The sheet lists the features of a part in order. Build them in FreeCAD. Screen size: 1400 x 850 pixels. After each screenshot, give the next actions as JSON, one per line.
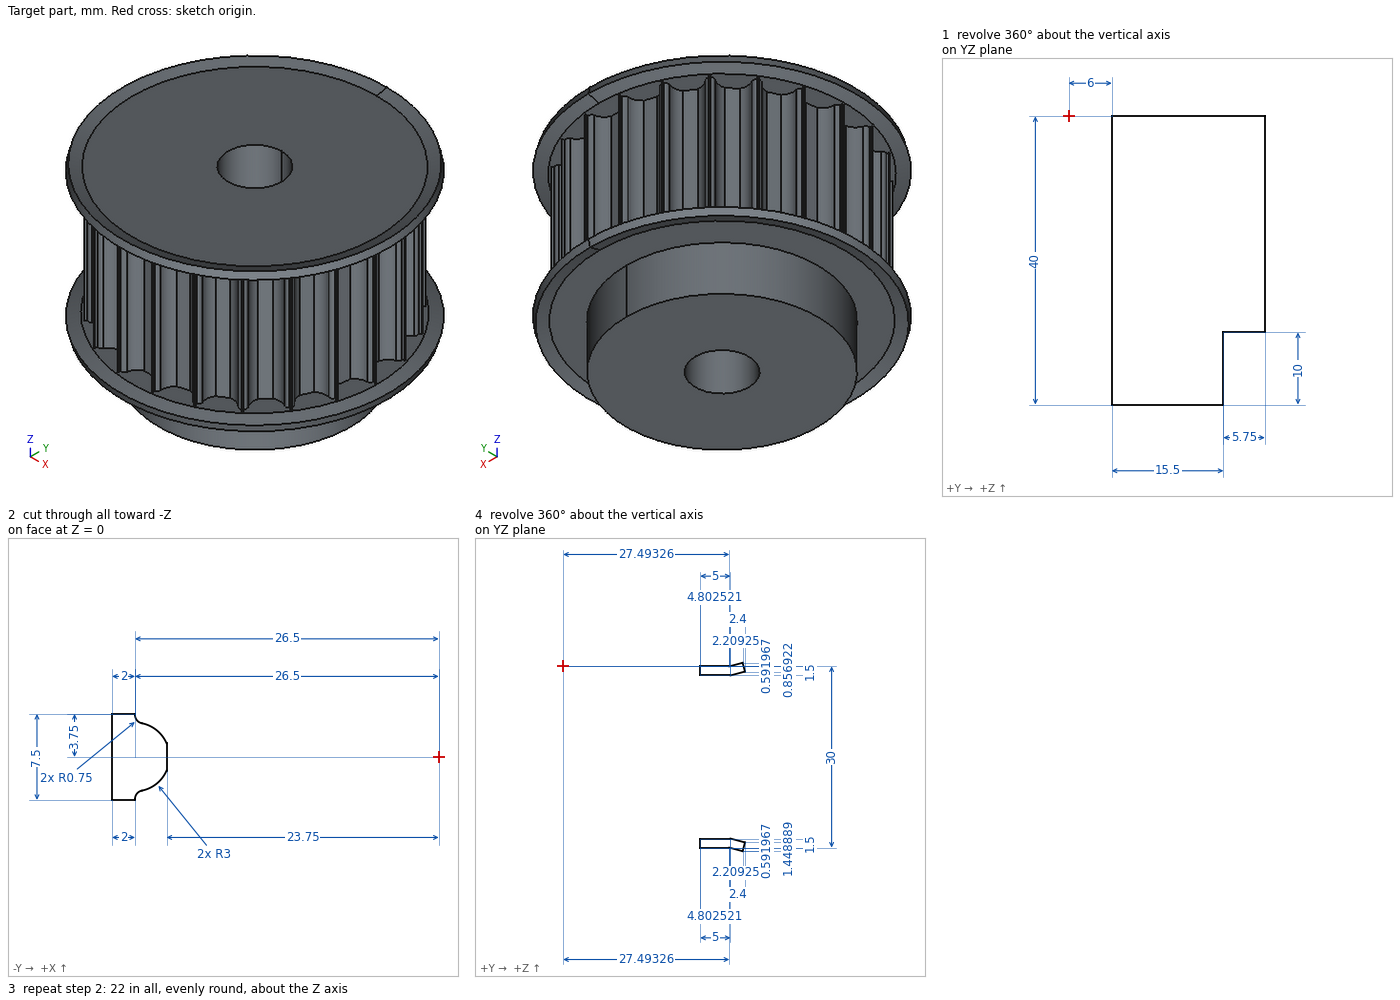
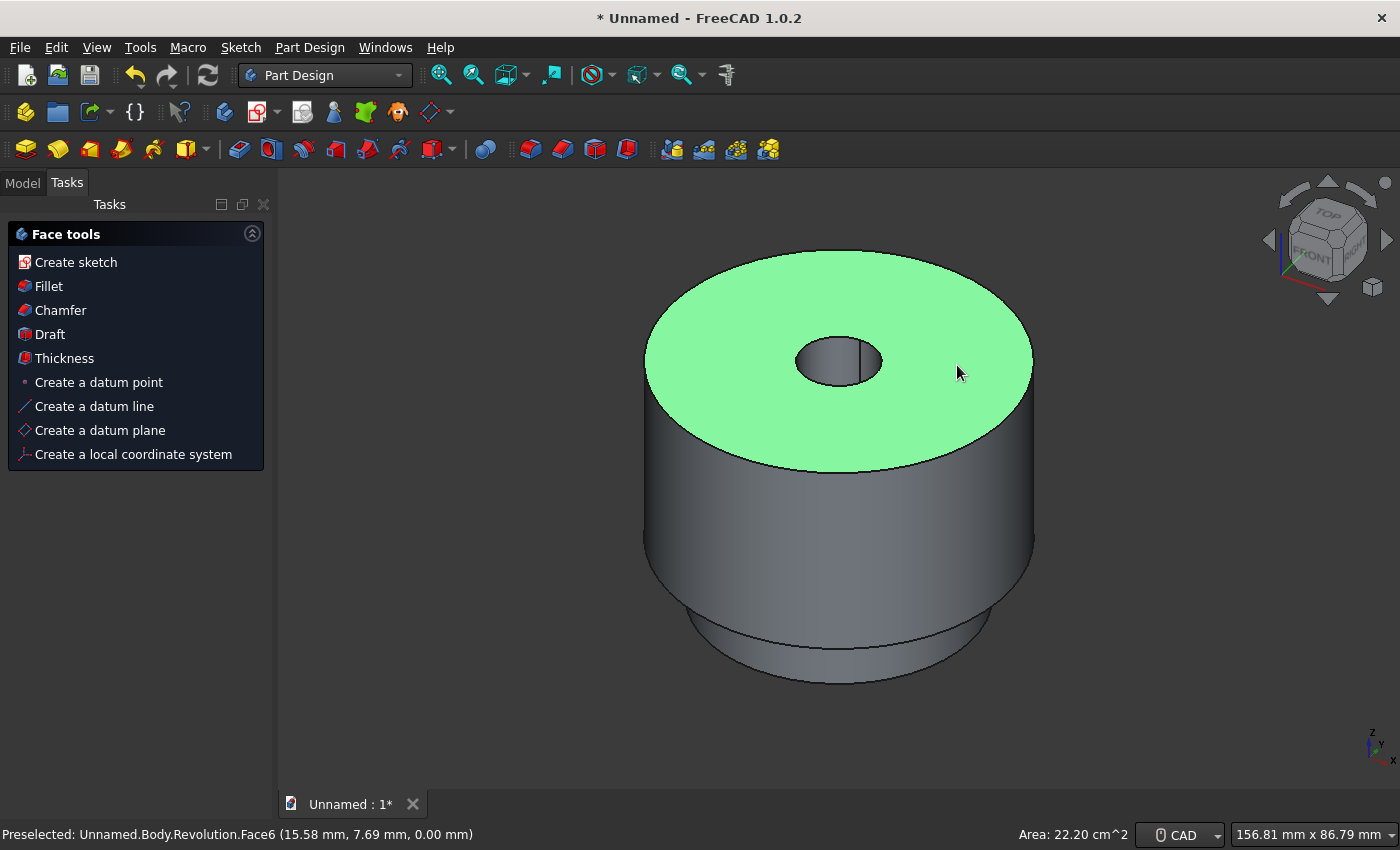
{"action": "left_click", "coordinate": [258, 112]}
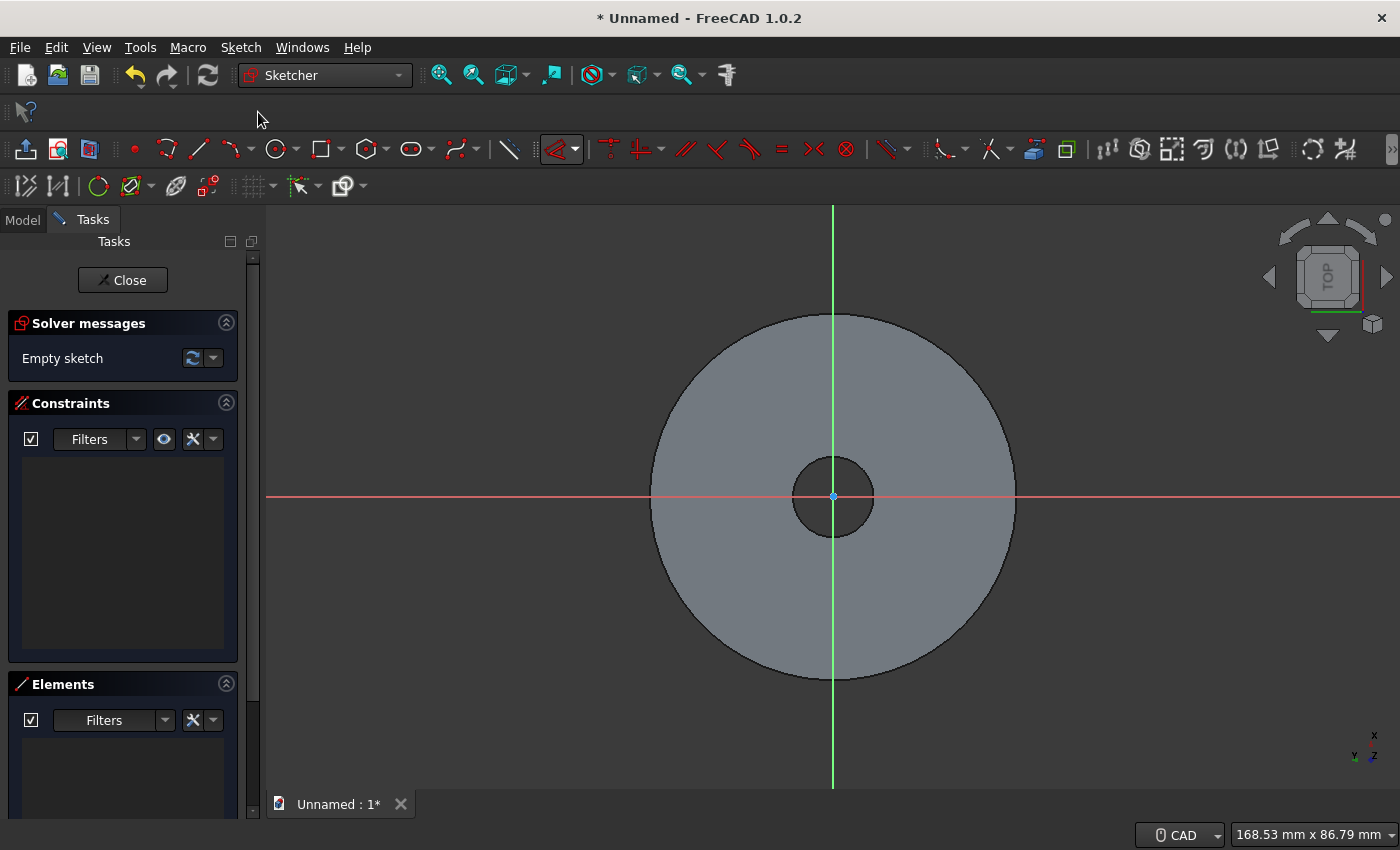
{"action": "scroll", "coordinate": [641, 497], "scroll_direction": "up", "scroll_amount": 10}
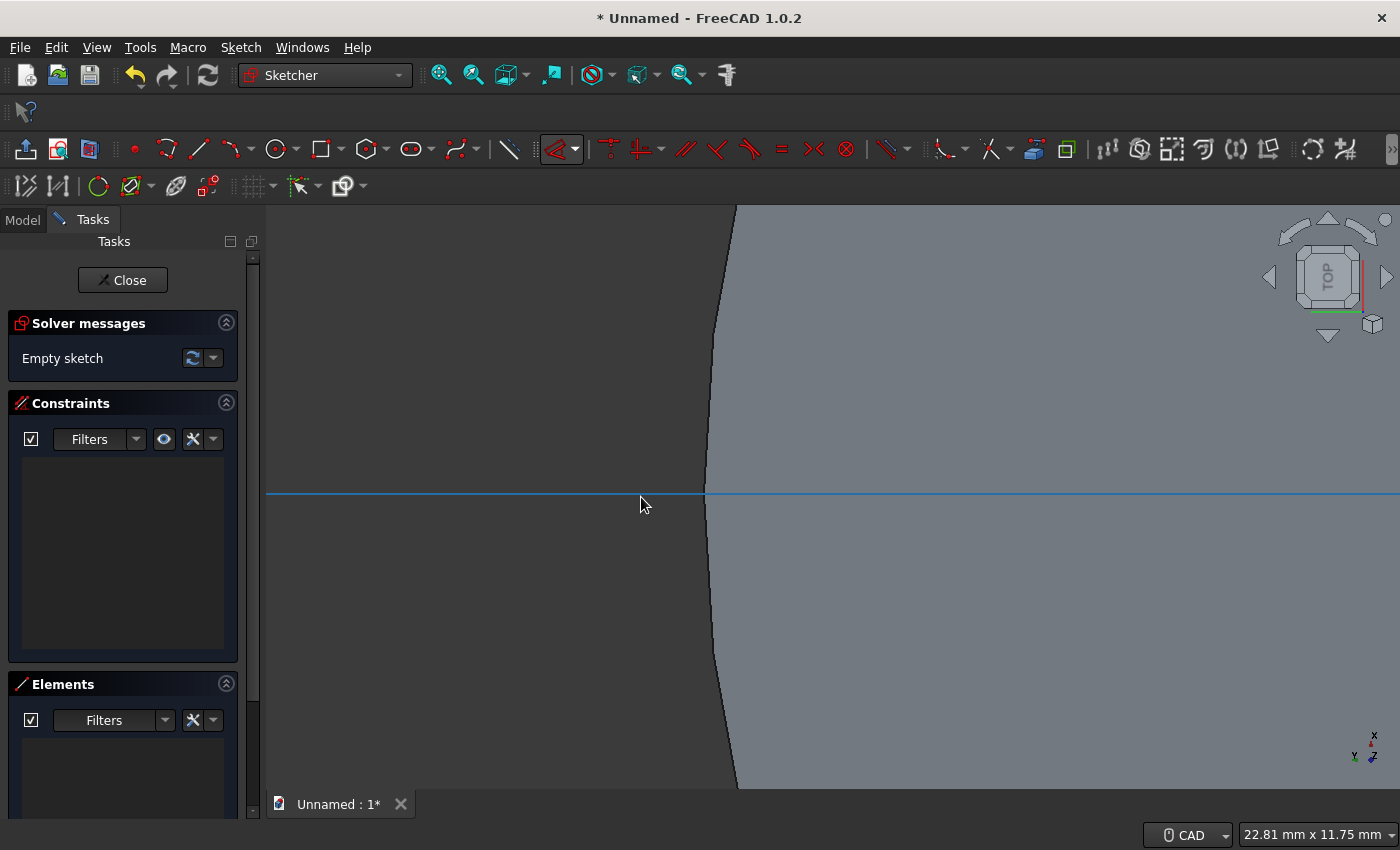
{"action": "left_click", "coordinate": [168, 150]}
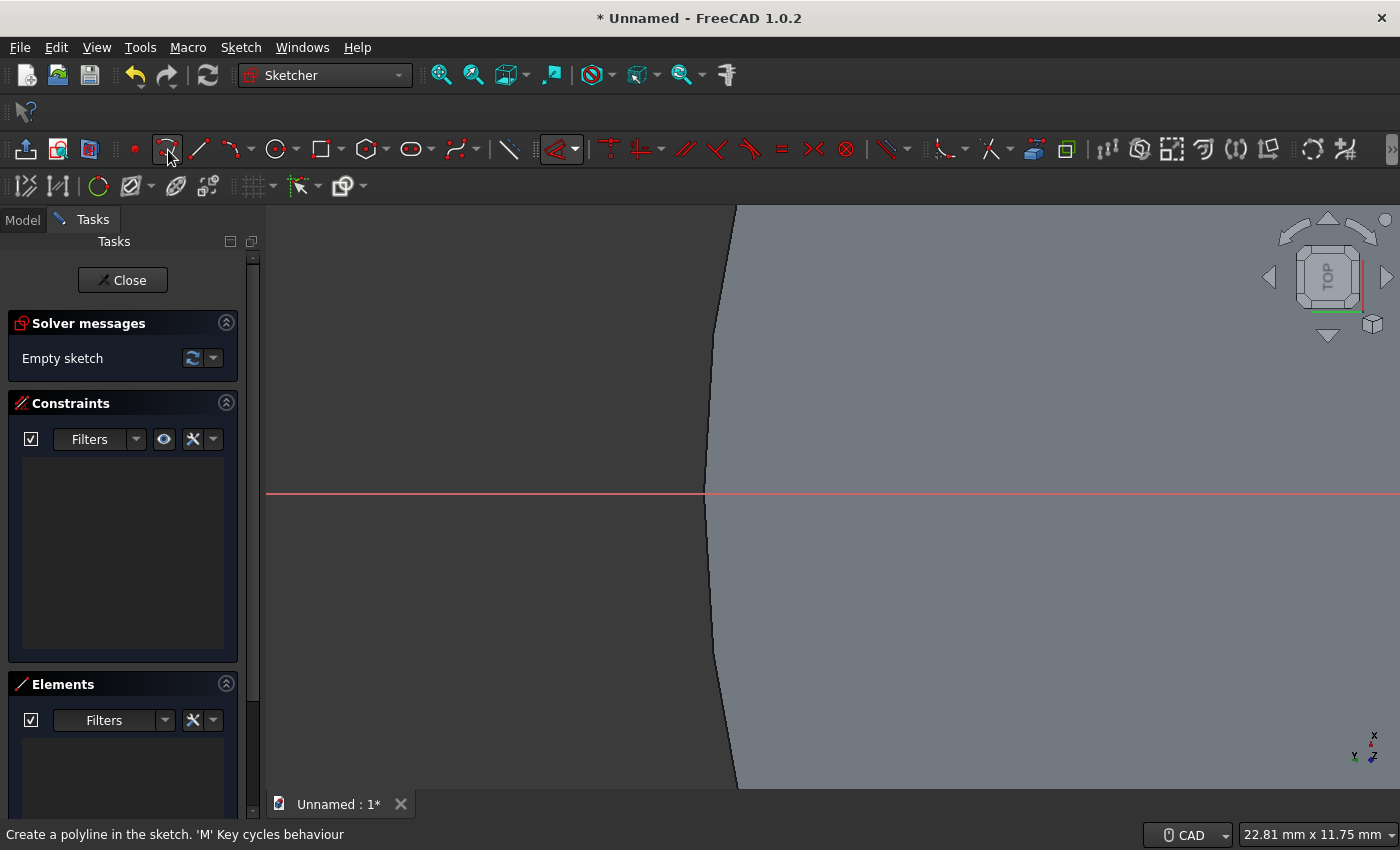
{"action": "left_click", "coordinate": [741, 311]}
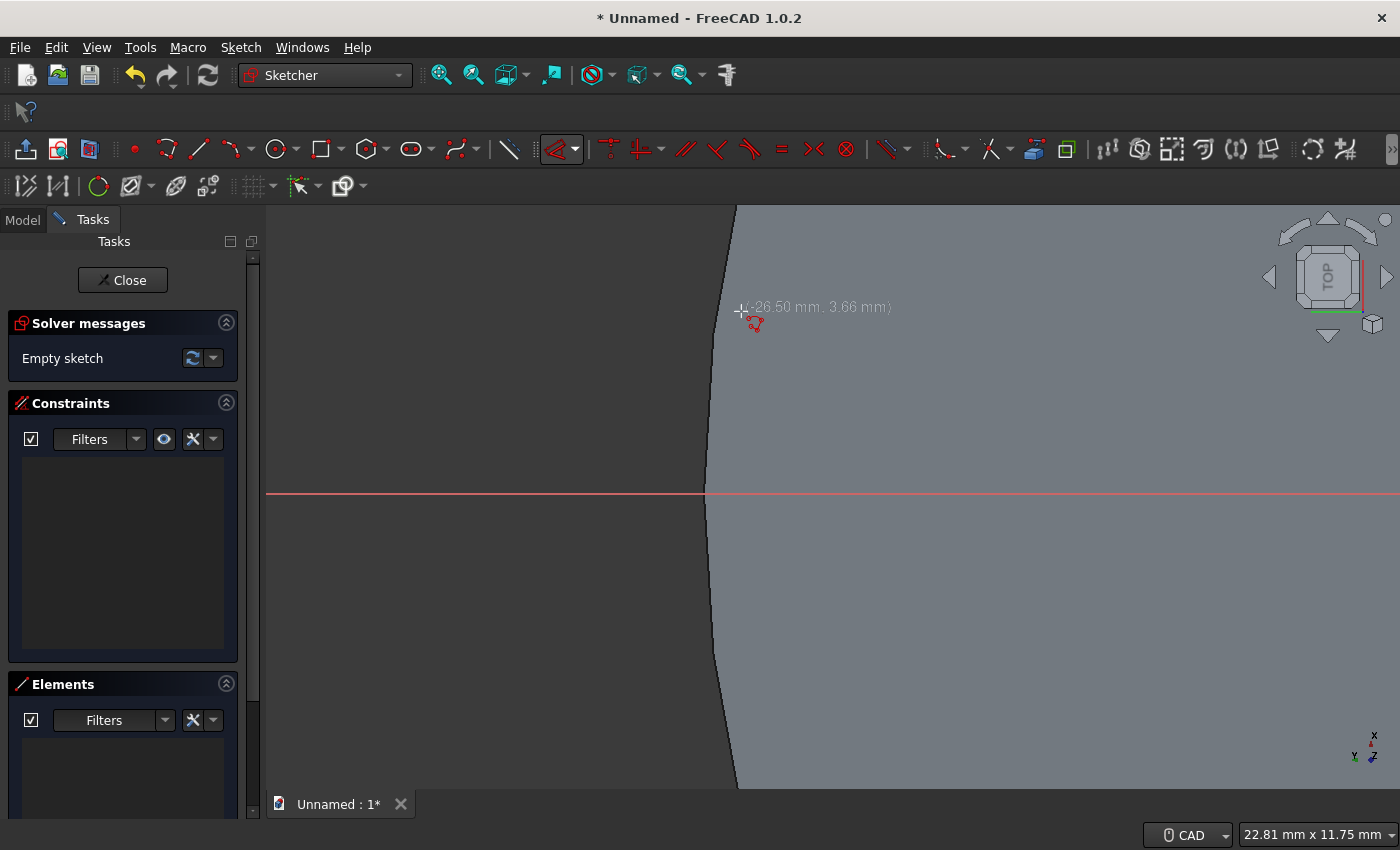
{"action": "scroll", "coordinate": [741, 307], "scroll_direction": "up", "scroll_amount": 8}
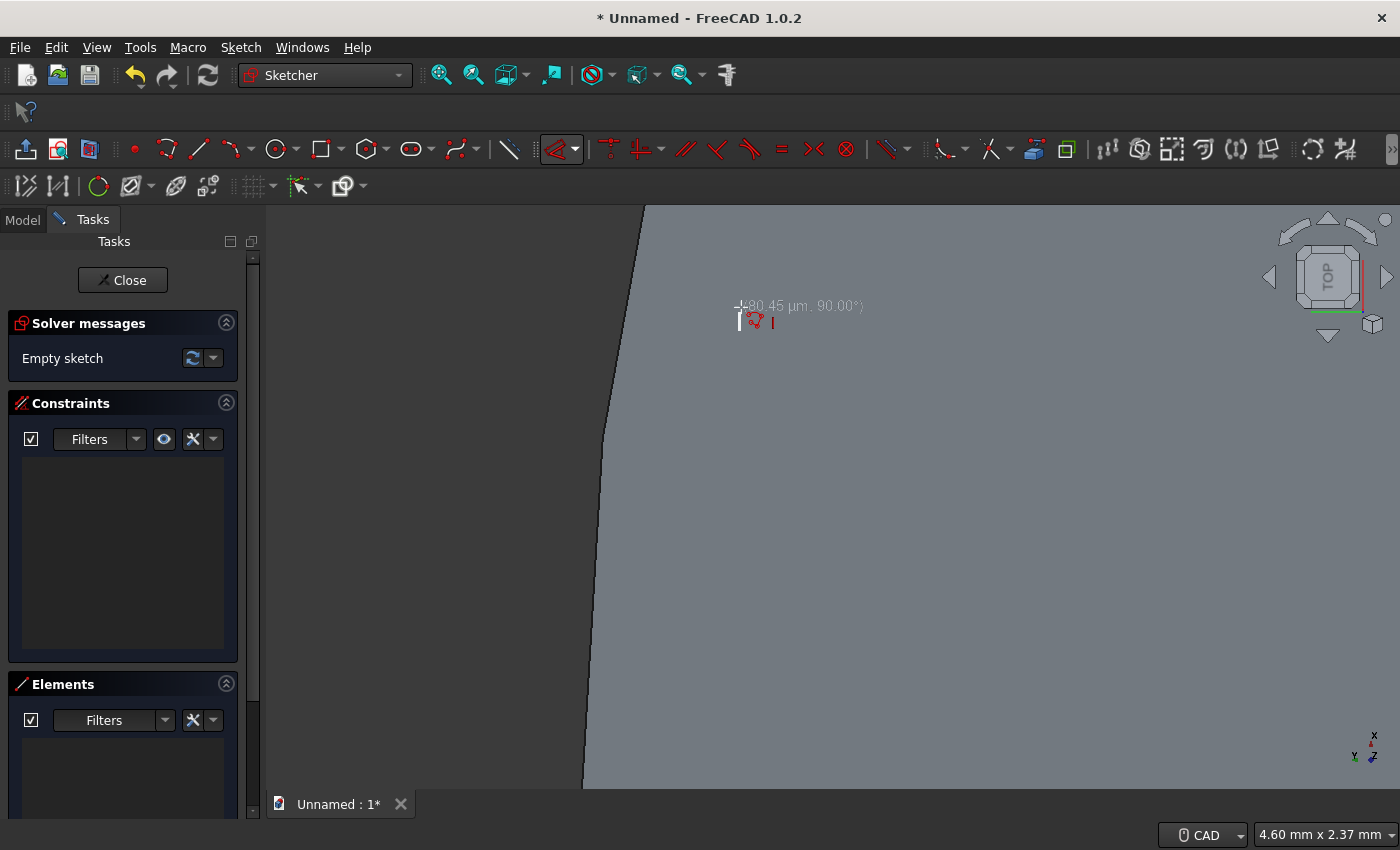
{"action": "left_click", "coordinate": [739, 308]}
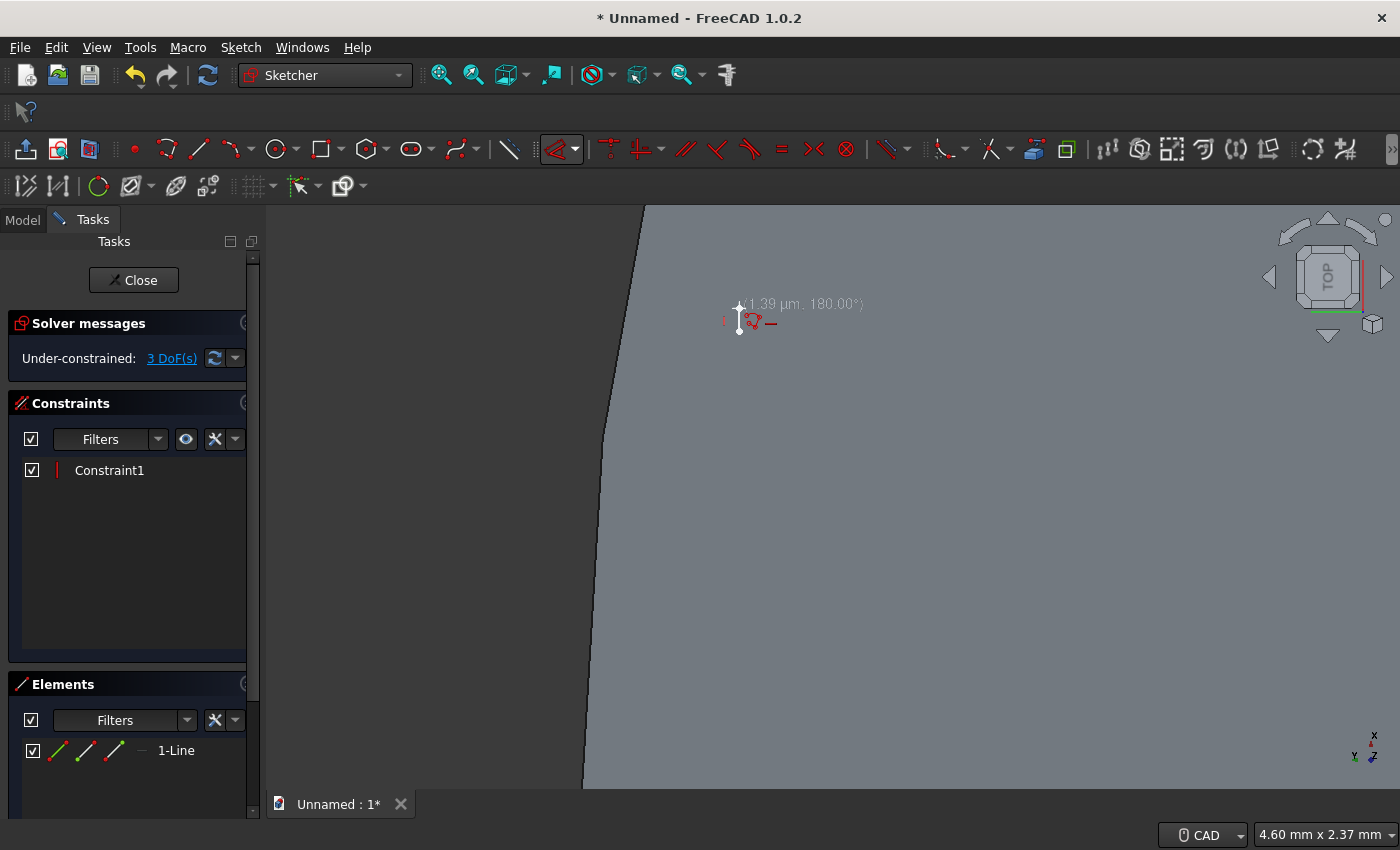
{"action": "scroll", "coordinate": [747, 311], "scroll_direction": "down", "scroll_amount": 8}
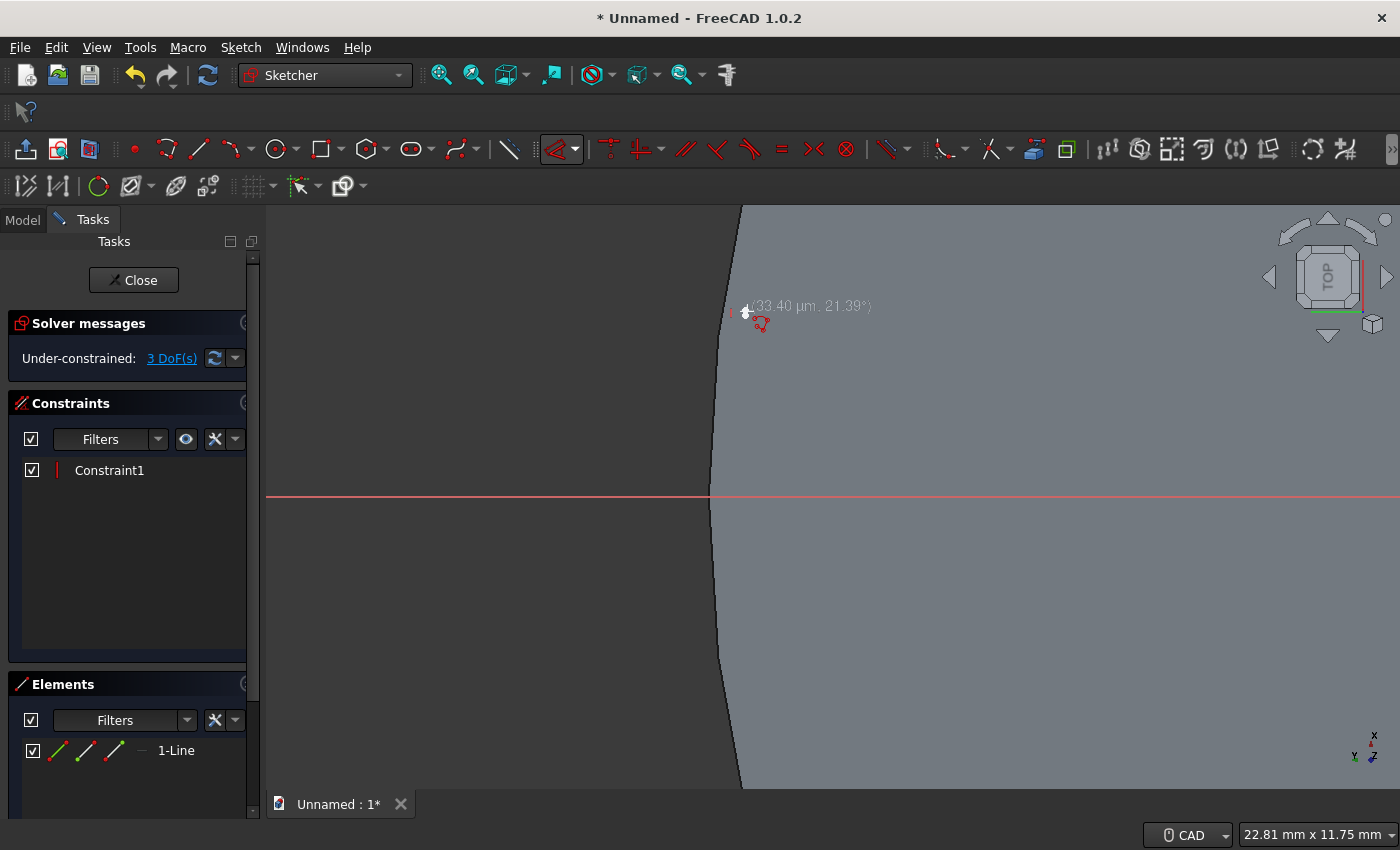
{"action": "left_click", "coordinate": [647, 311]}
{"action": "left_click", "coordinate": [647, 683]}
{"action": "left_click", "coordinate": [746, 683]}